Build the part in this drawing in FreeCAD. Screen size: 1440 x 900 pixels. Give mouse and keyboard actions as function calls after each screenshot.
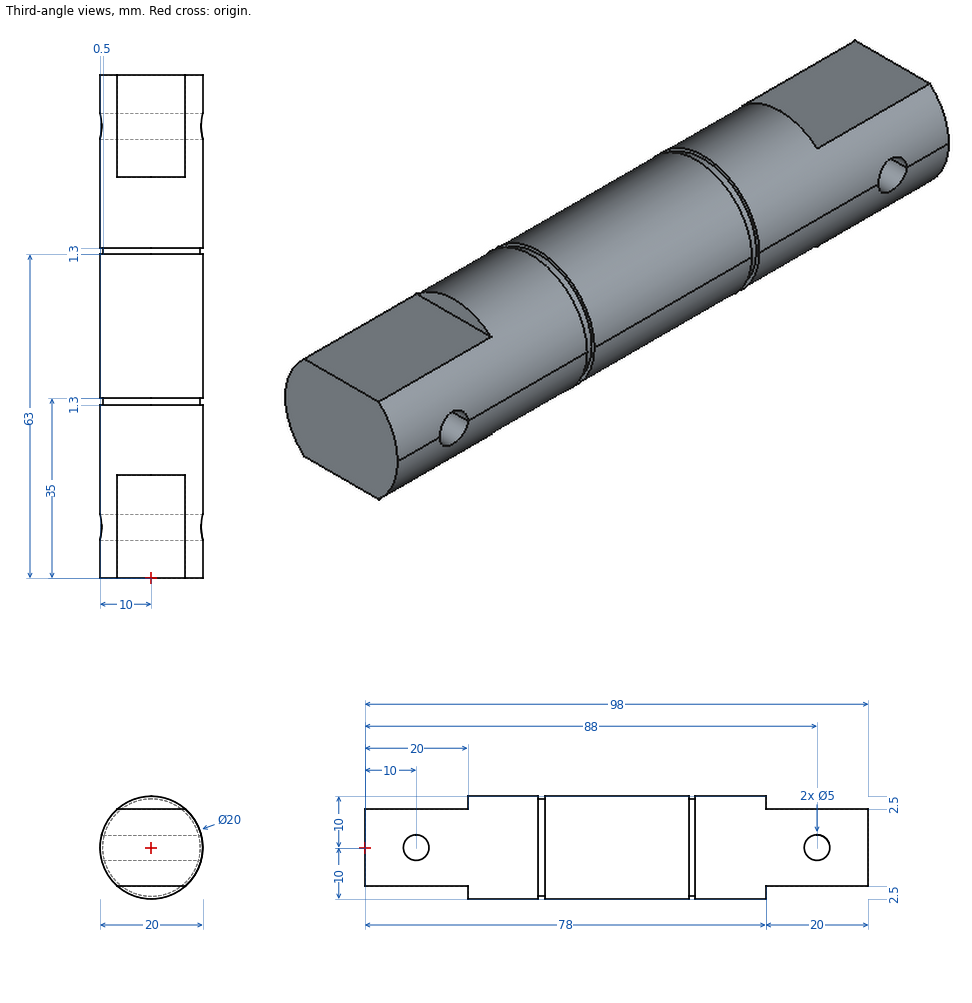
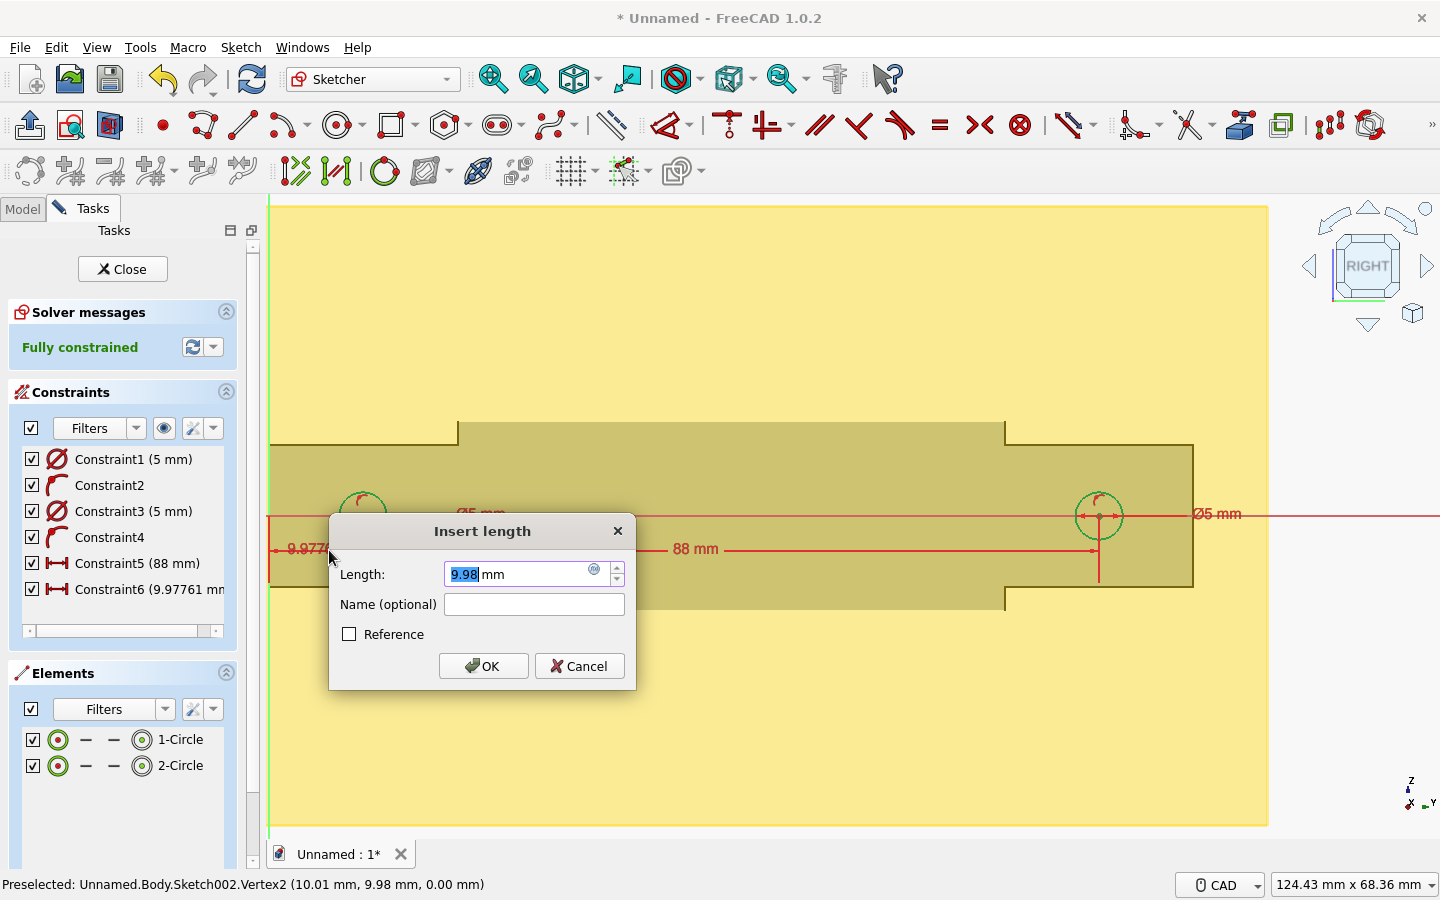
text(10)
key(Return)
key(Escape)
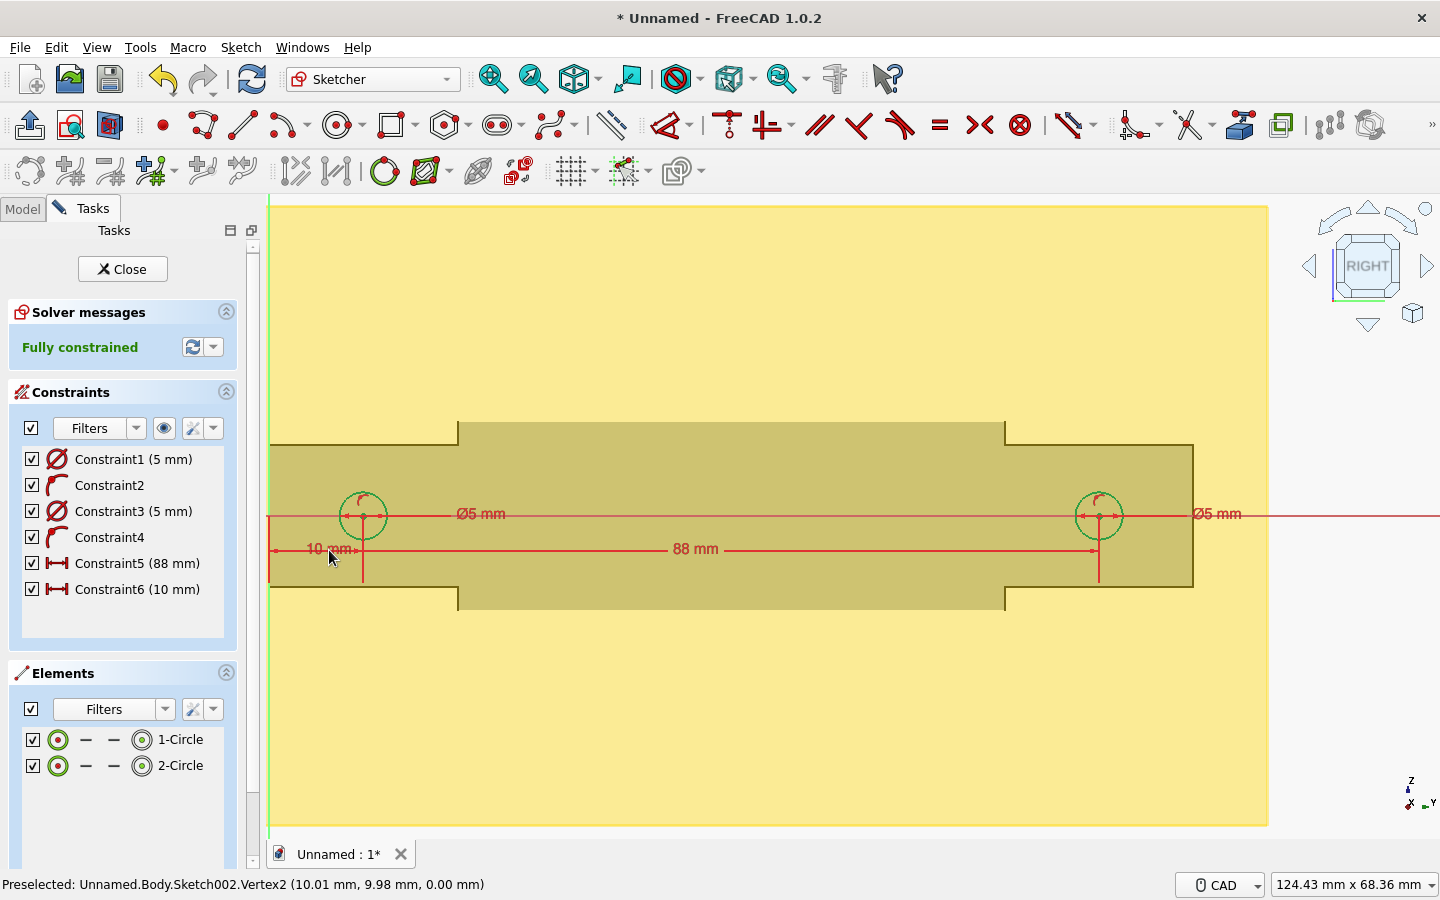
click(123, 269)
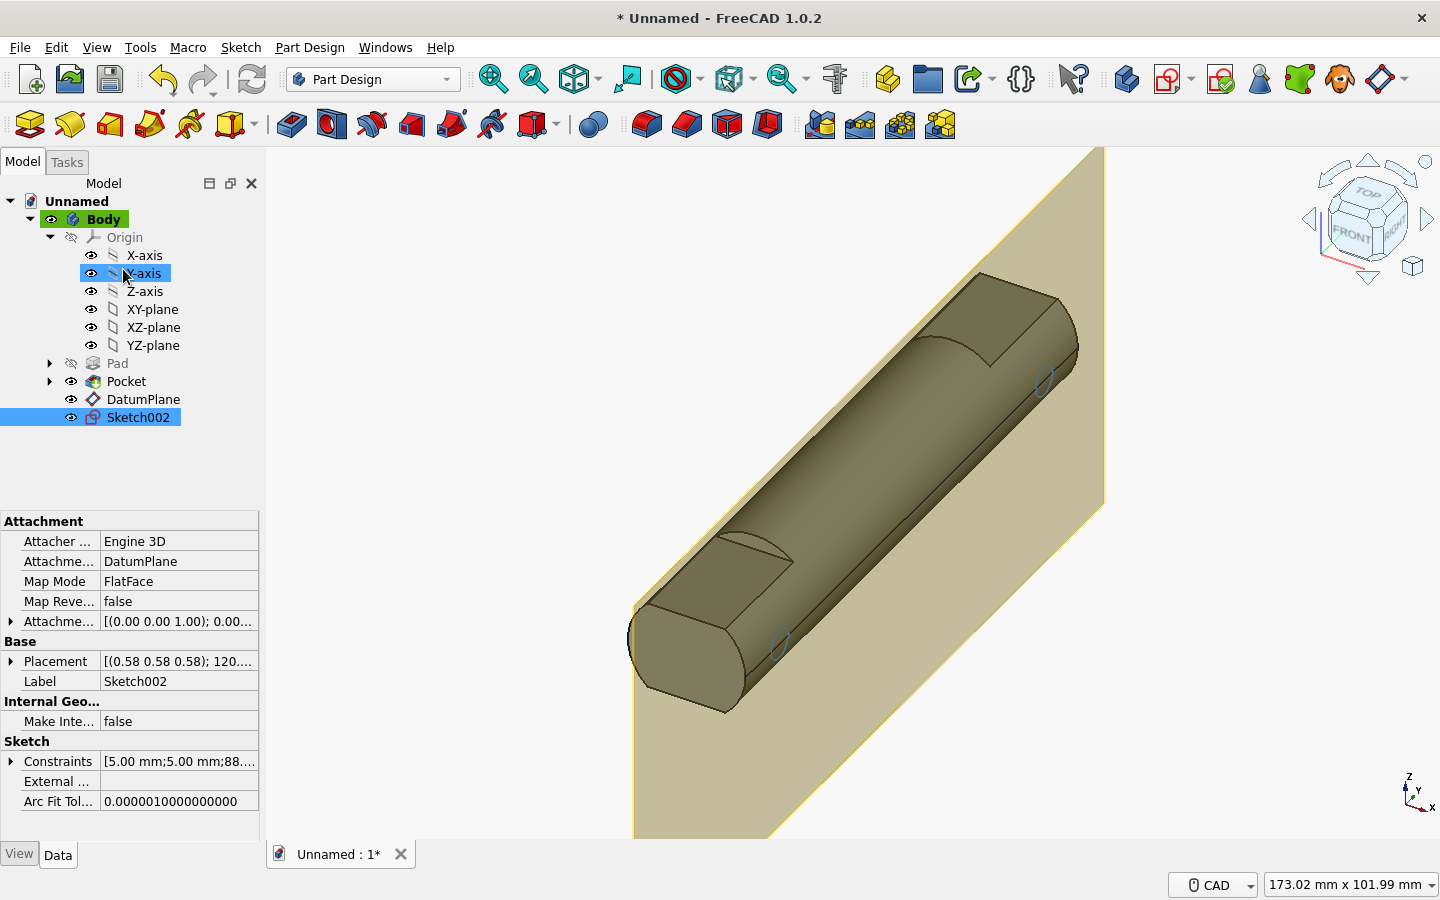
click(292, 124)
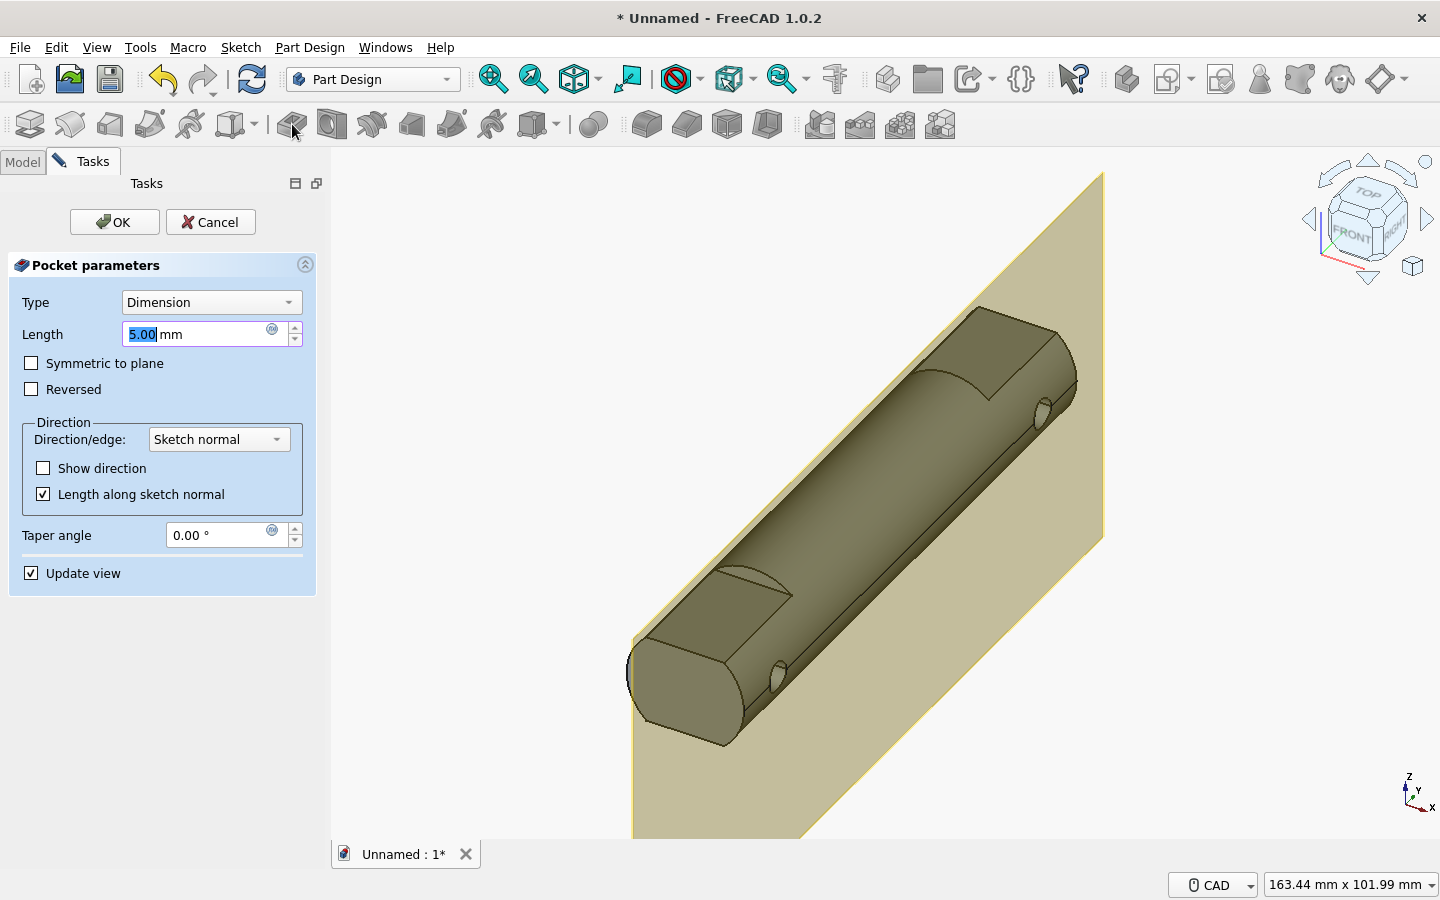
click(212, 302)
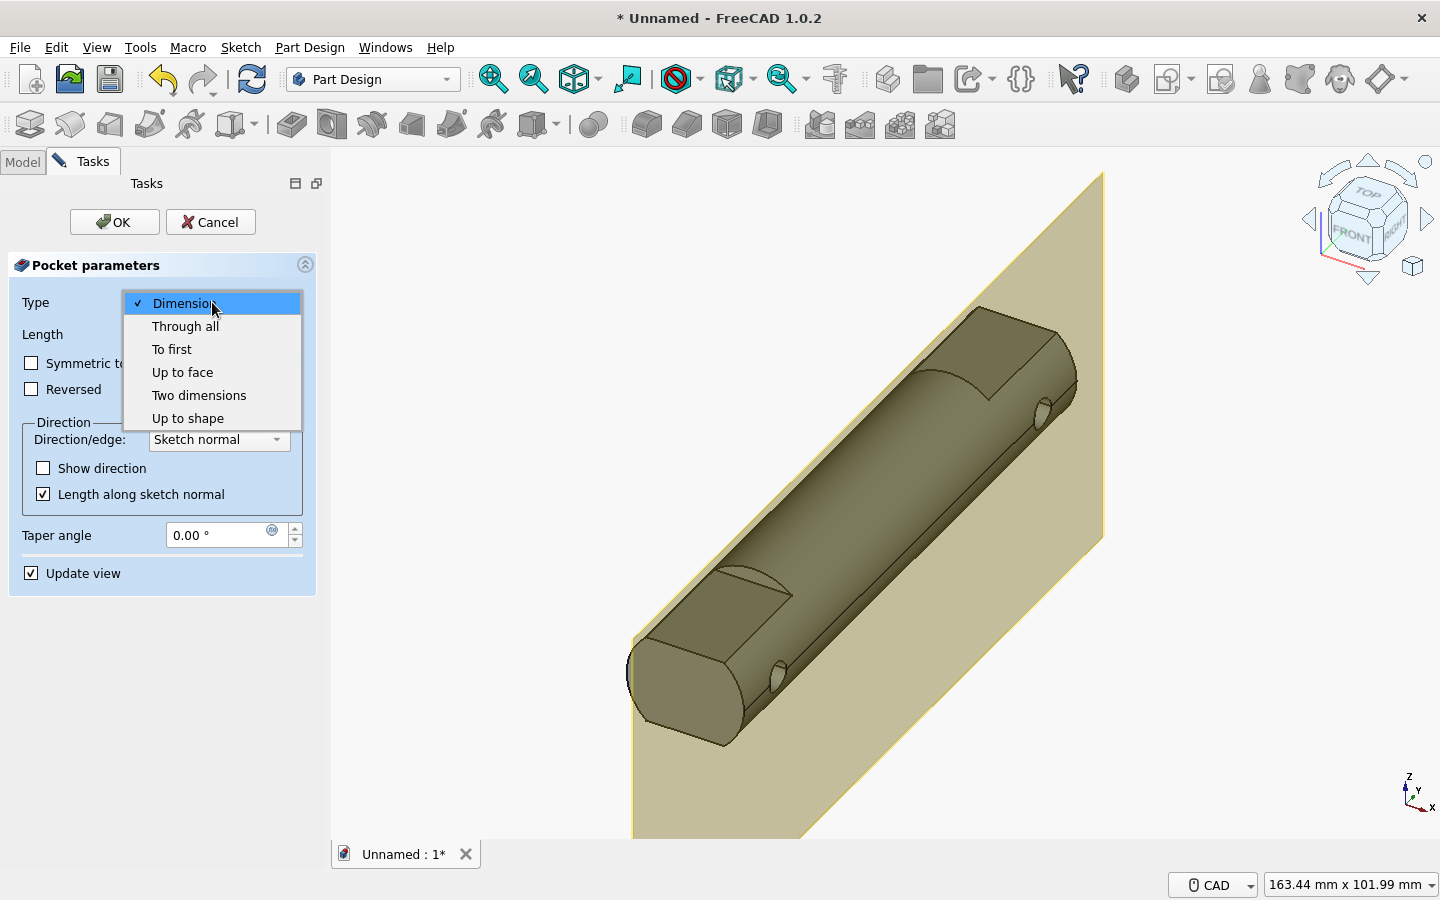
click(212, 326)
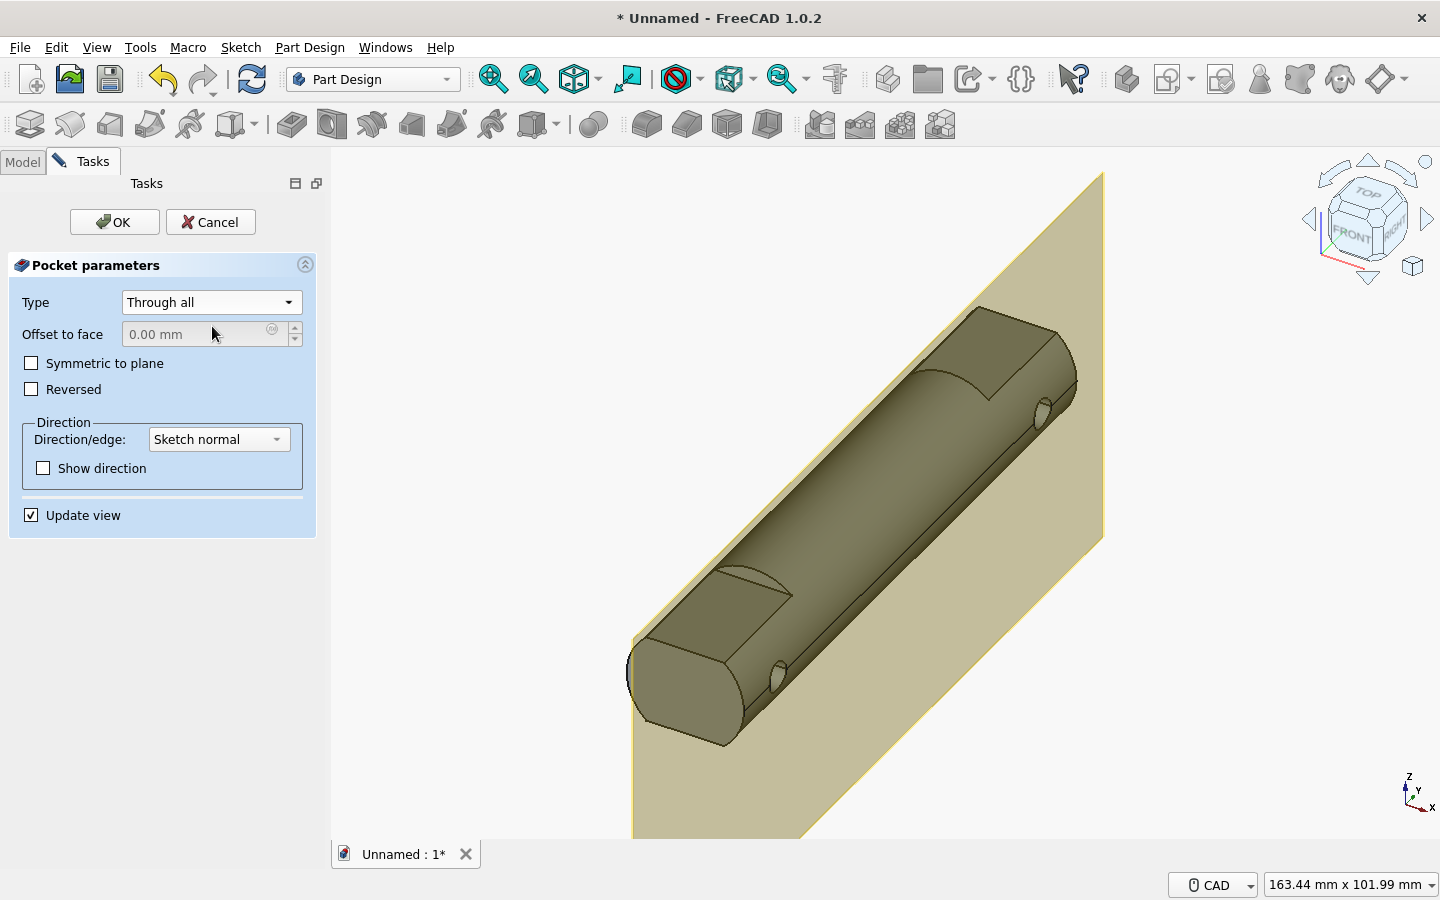
click(115, 222)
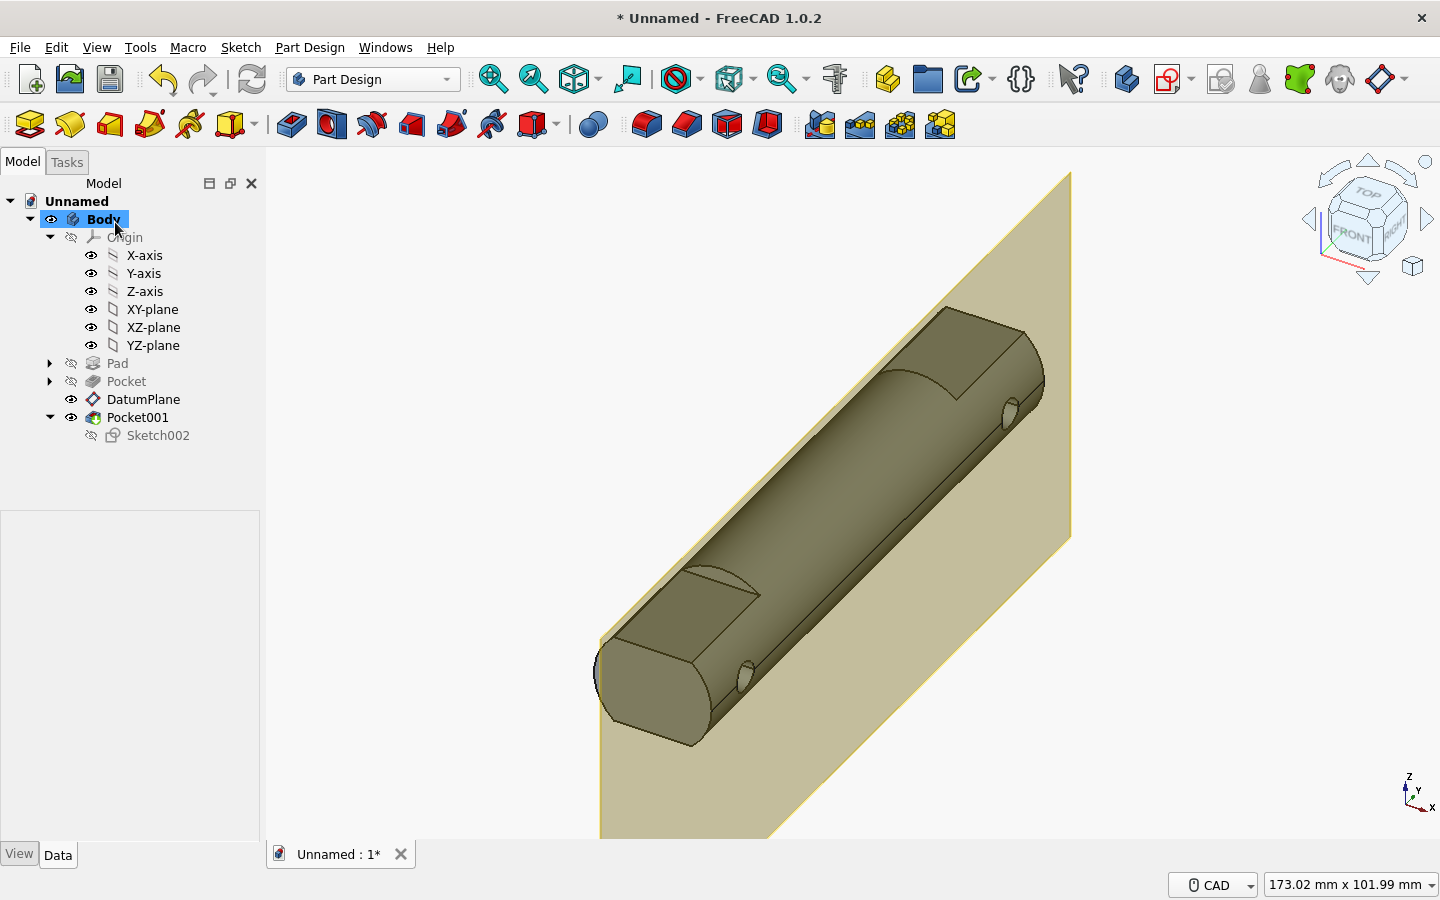
click(116, 399)
key(space)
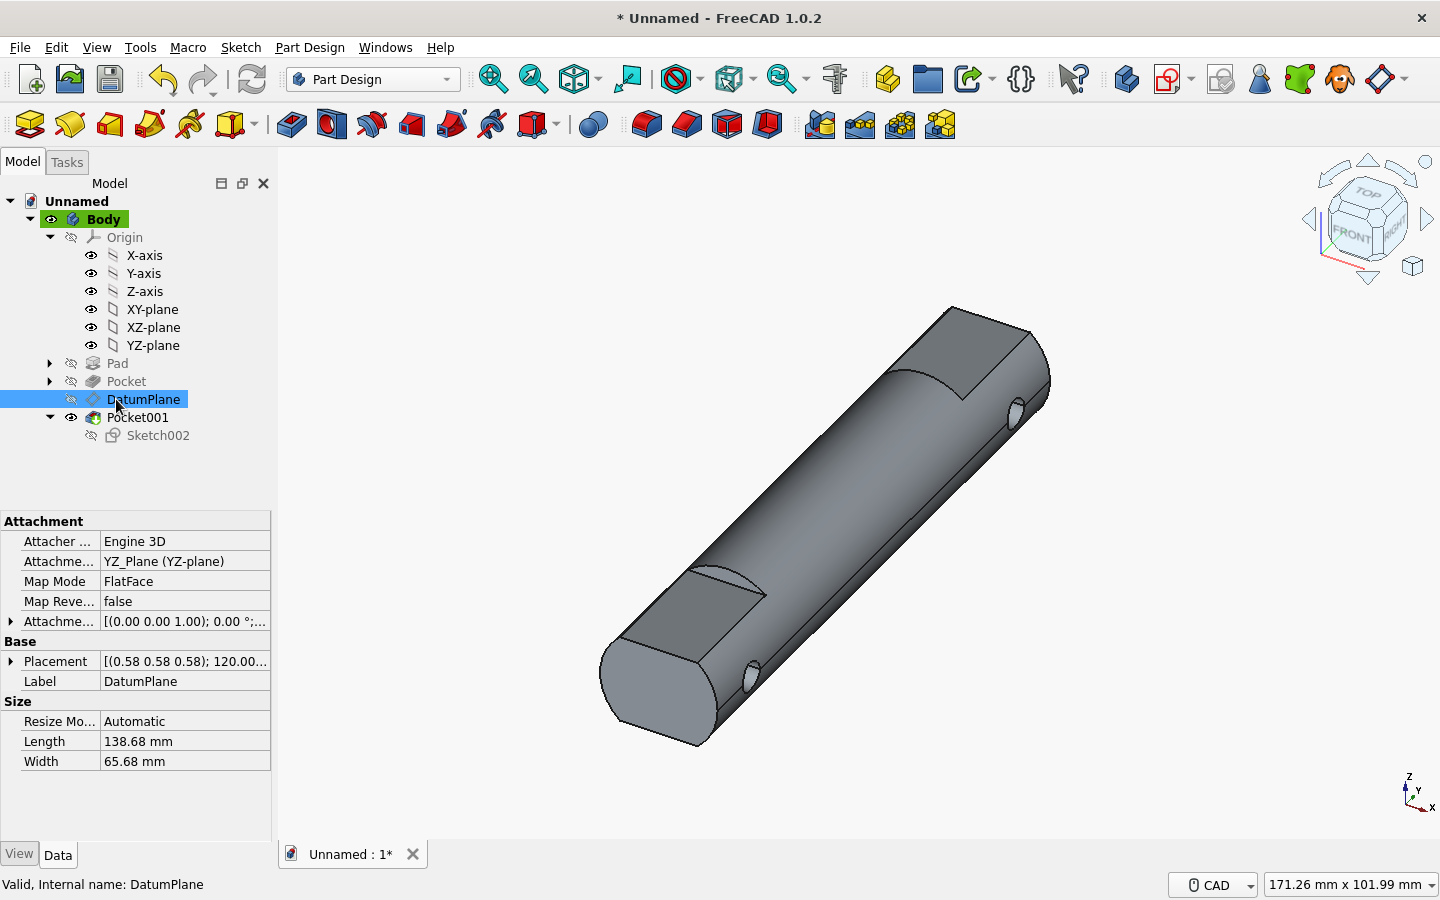
click(318, 799)